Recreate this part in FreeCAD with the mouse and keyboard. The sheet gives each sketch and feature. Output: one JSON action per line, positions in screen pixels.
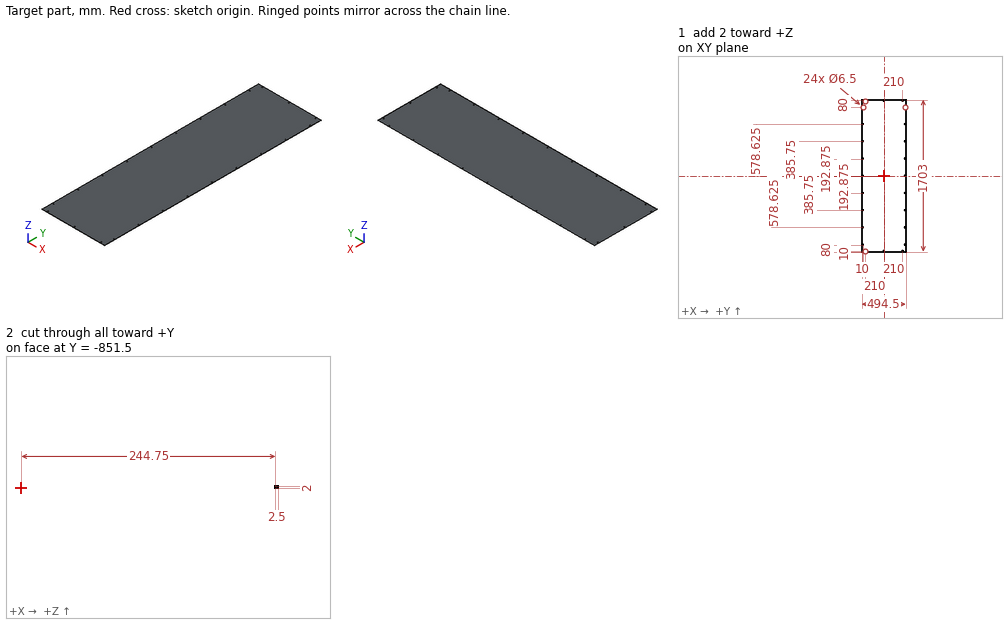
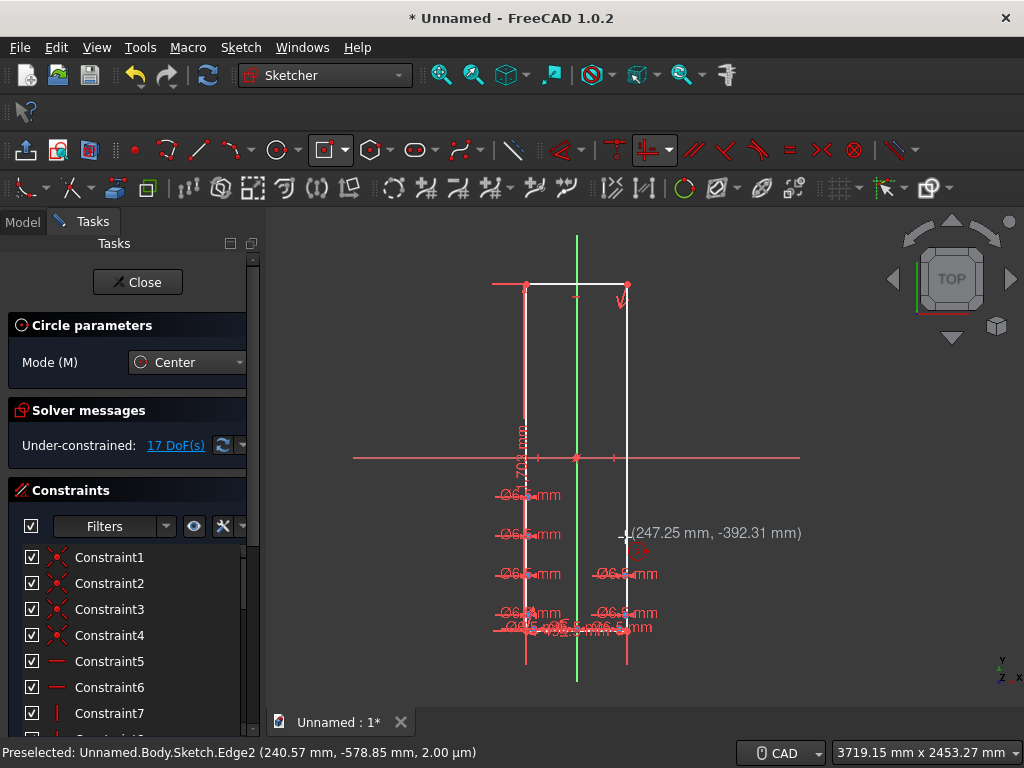
{"action": "scroll", "coordinate": [625, 536], "scroll_direction": "up", "scroll_amount": 11}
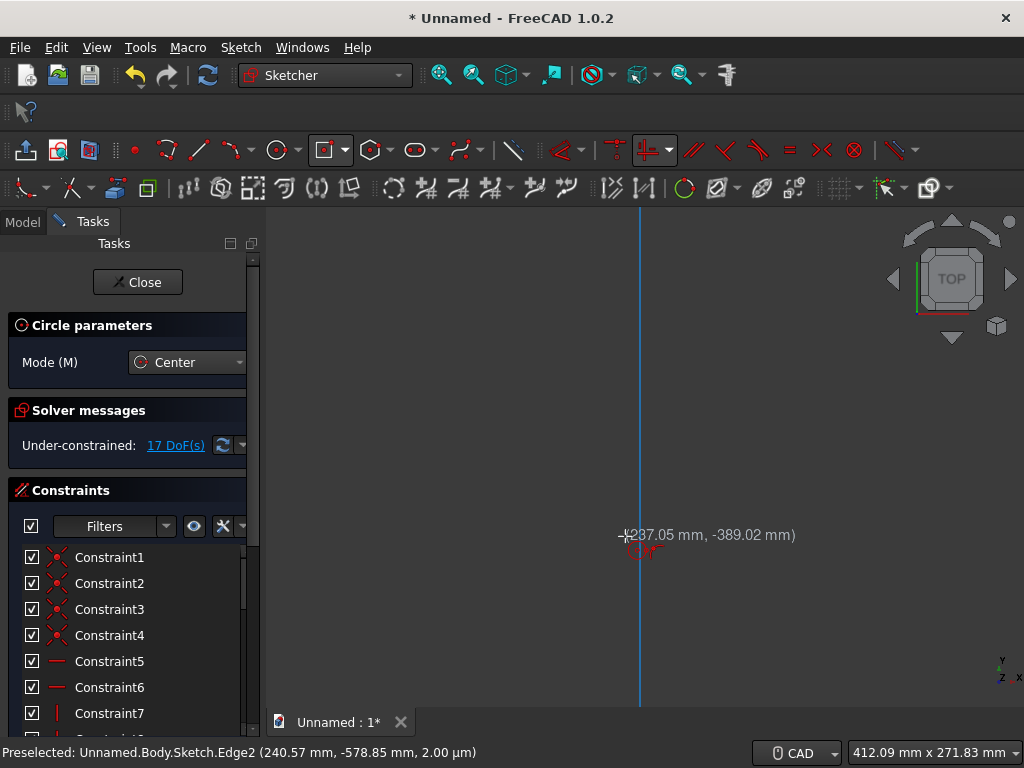
{"action": "left_click", "coordinate": [622, 534]}
{"action": "mouse_move", "coordinate": [626, 529]}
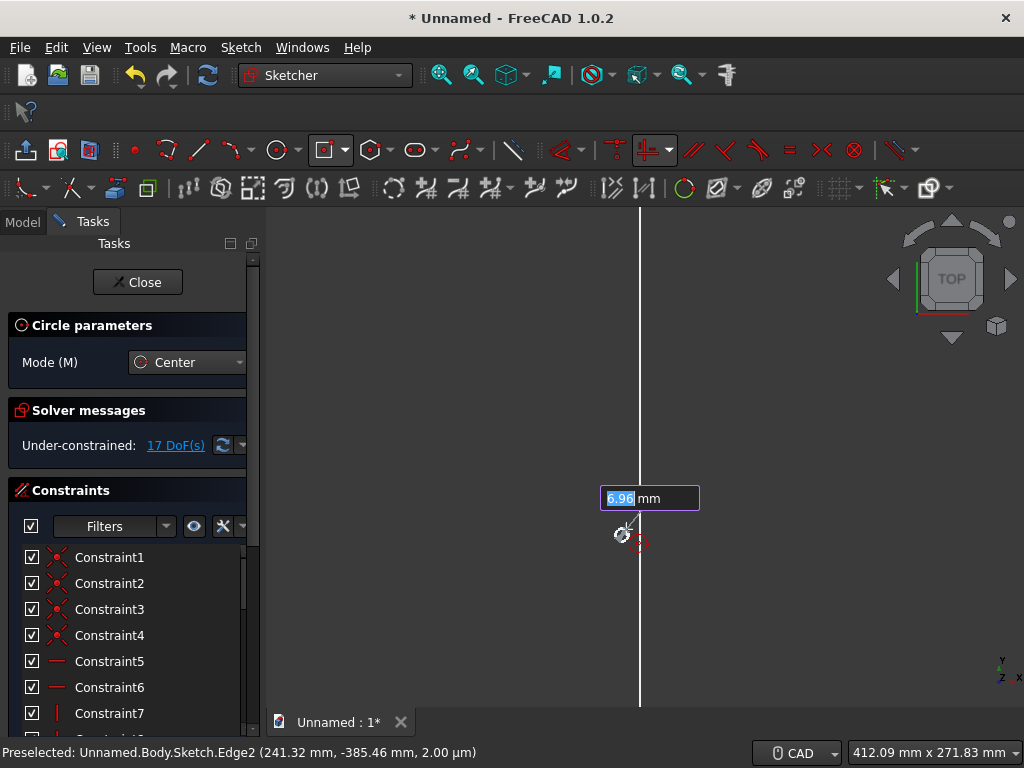
{"action": "type", "text": "6.5"}
{"action": "key", "text": "Return"}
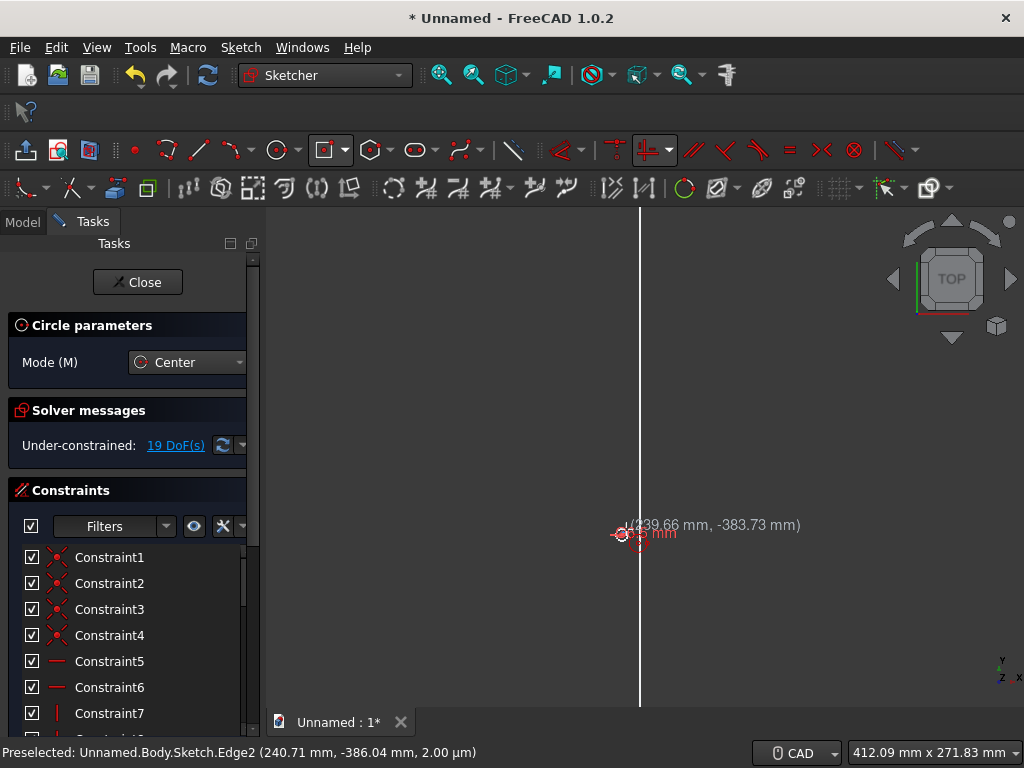
{"action": "scroll", "coordinate": [616, 520], "scroll_direction": "down", "scroll_amount": 12}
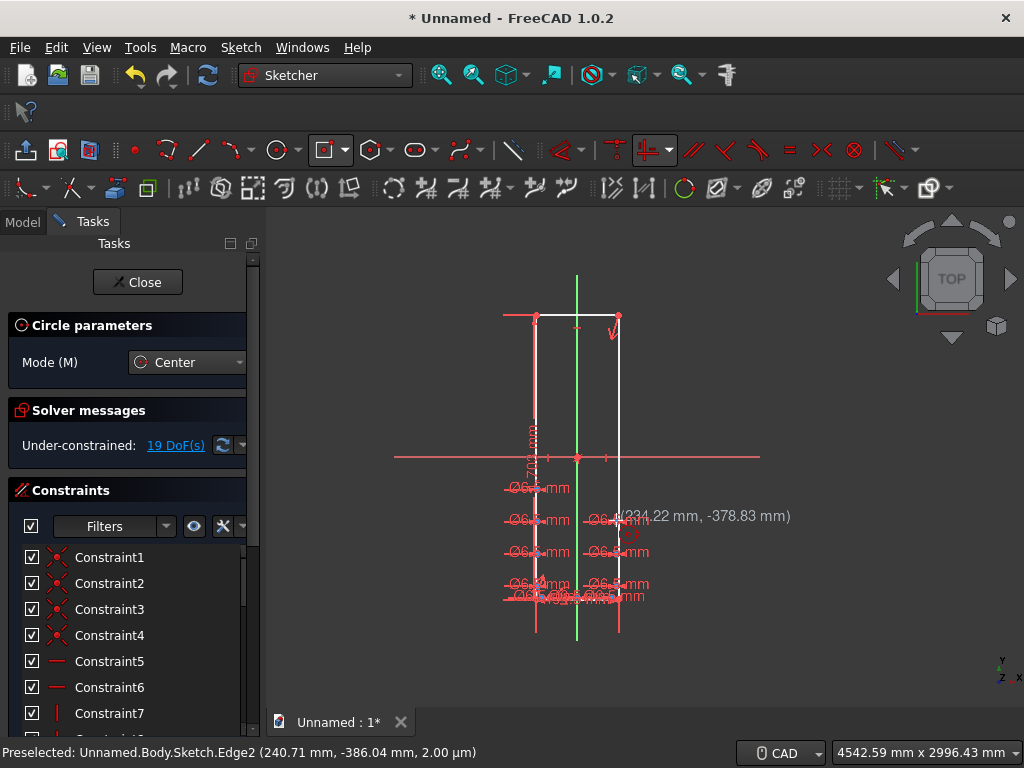
{"action": "scroll", "coordinate": [617, 490], "scroll_direction": "up", "scroll_amount": 19}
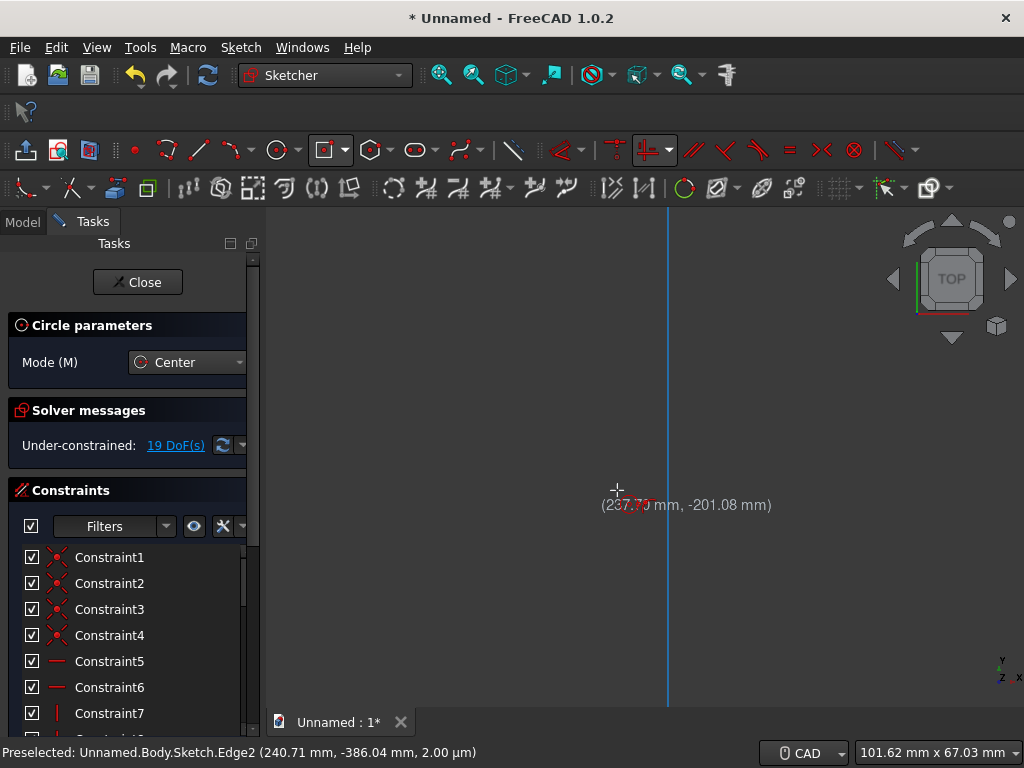
{"action": "scroll", "coordinate": [626, 498], "scroll_direction": "down", "scroll_amount": 18}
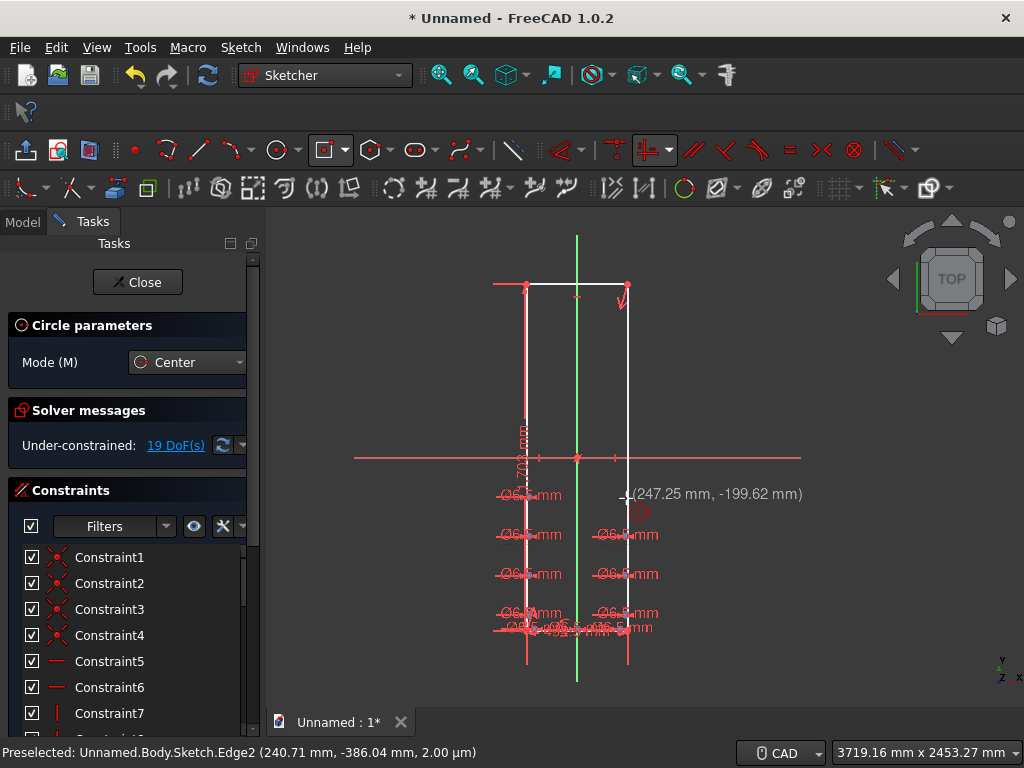
{"action": "scroll", "coordinate": [626, 497], "scroll_direction": "up", "scroll_amount": 11}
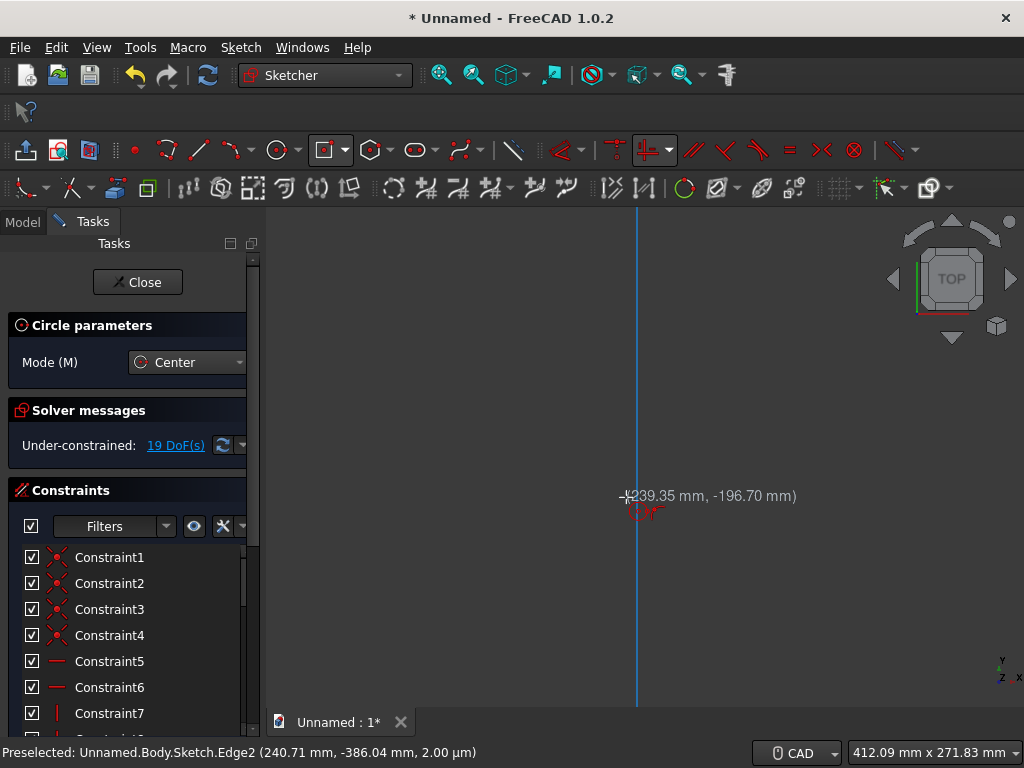
{"action": "left_click", "coordinate": [618, 494]}
{"action": "mouse_move", "coordinate": [623, 490]}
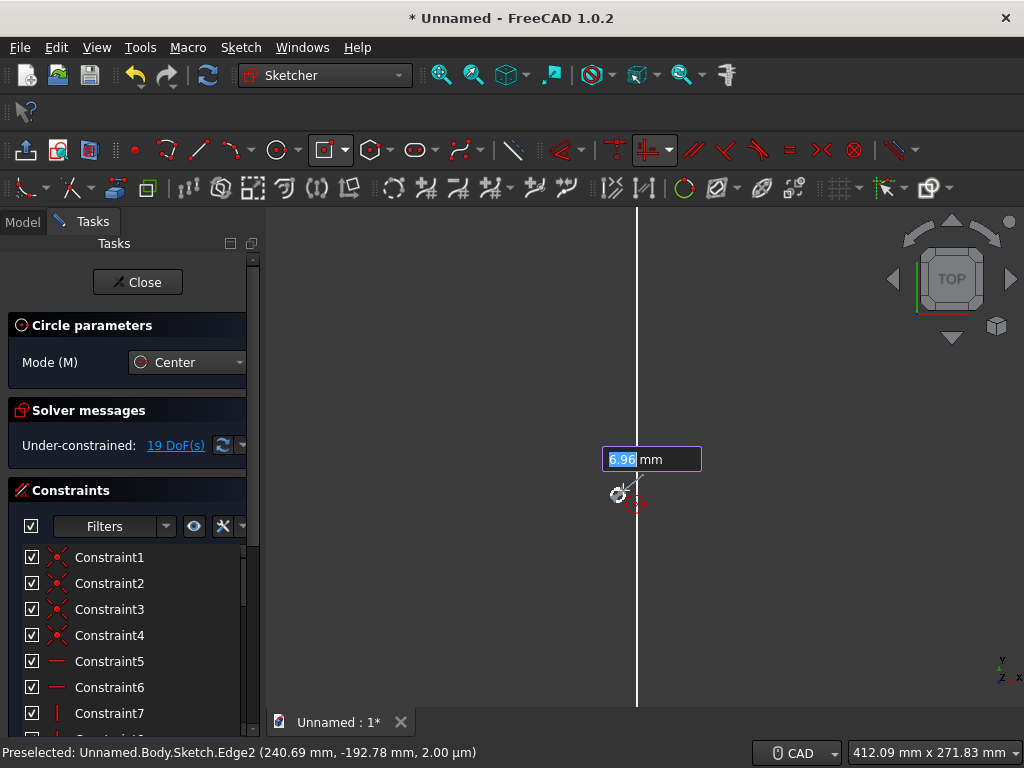
{"action": "type", "text": "6.5"}
{"action": "key", "text": "Return"}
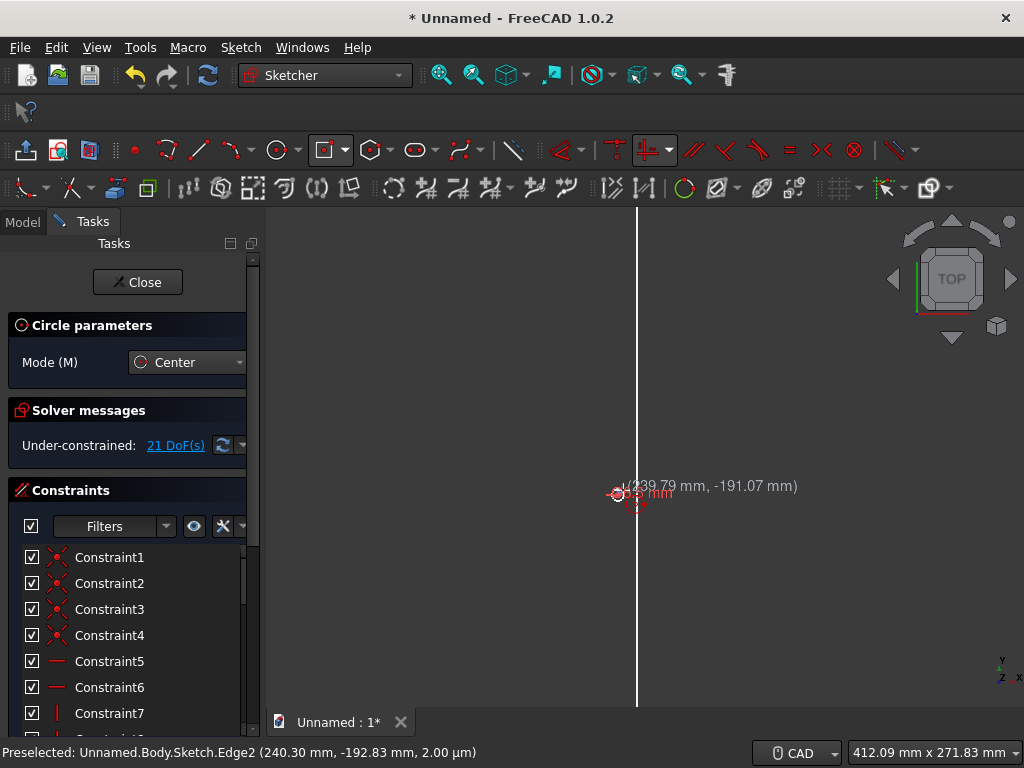
{"action": "scroll", "coordinate": [616, 489], "scroll_direction": "down", "scroll_amount": 12}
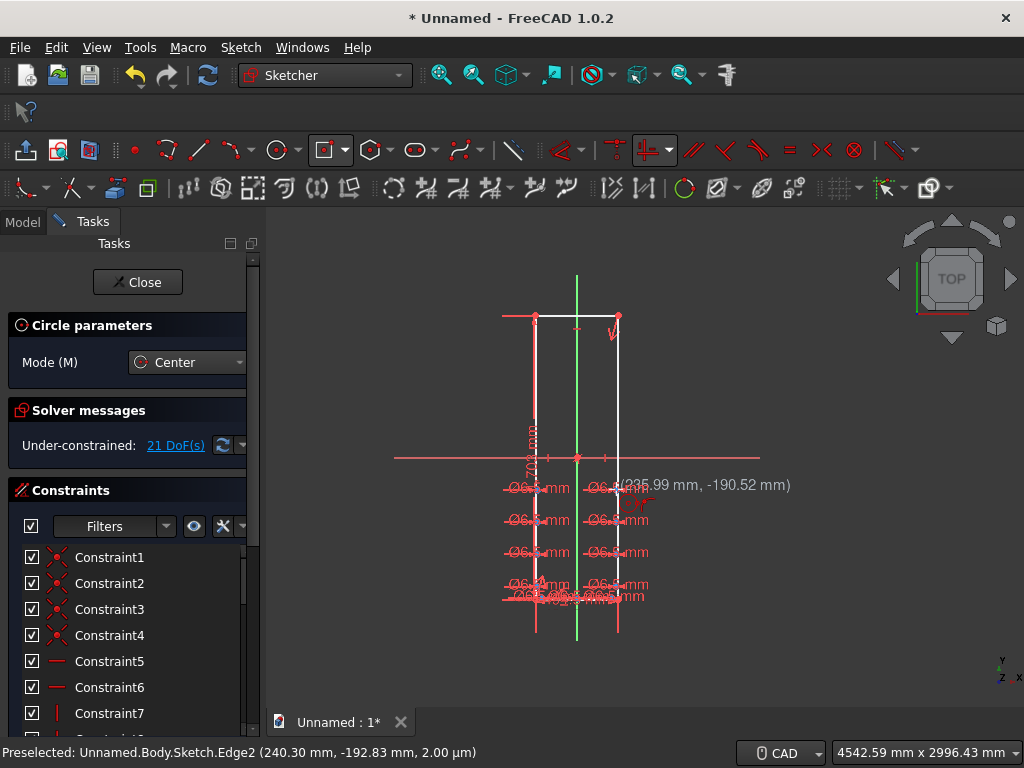
{"action": "scroll", "coordinate": [537, 458], "scroll_direction": "up", "scroll_amount": 19}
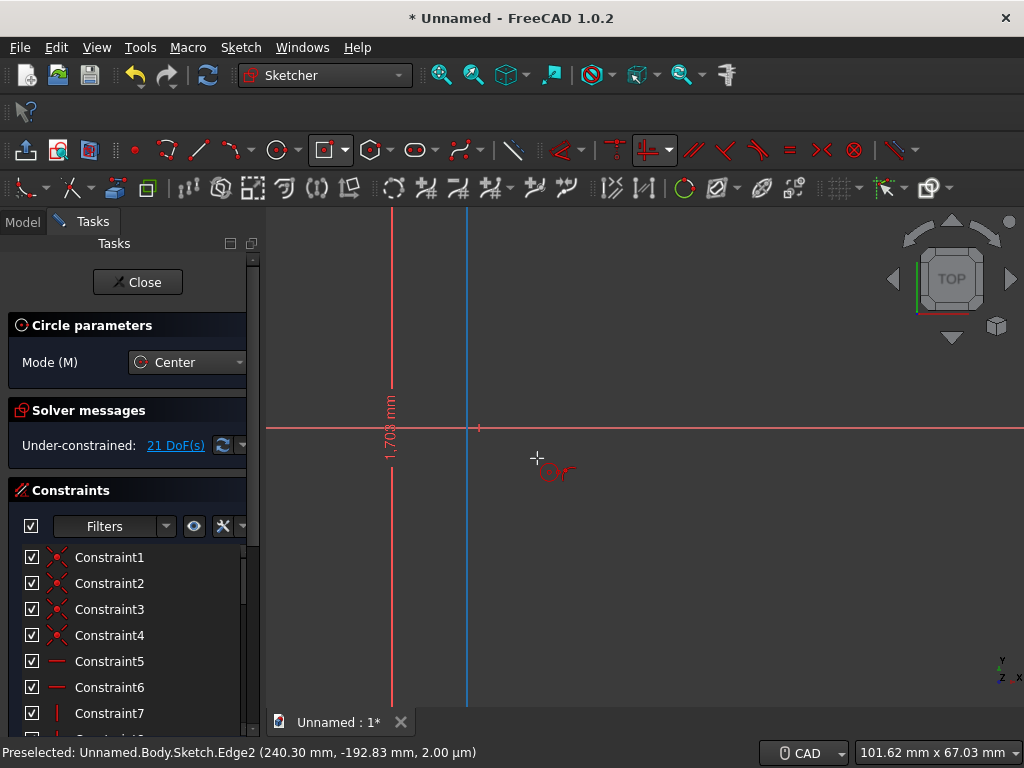
{"action": "scroll", "coordinate": [528, 458], "scroll_direction": "down", "scroll_amount": 18}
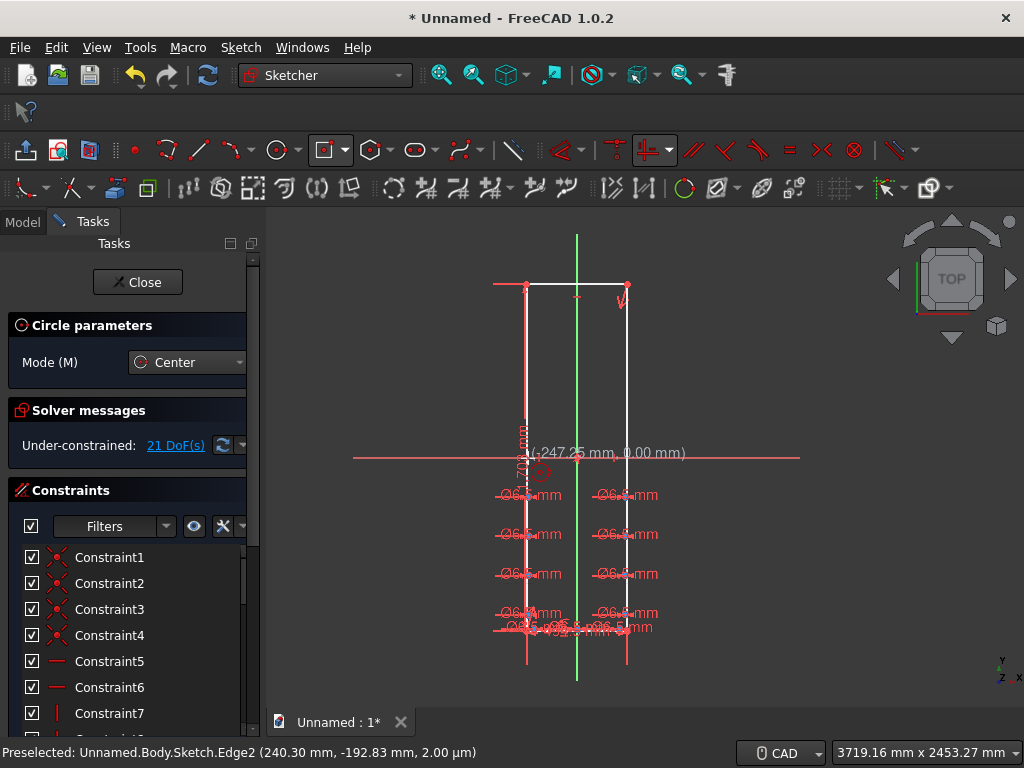
{"action": "scroll", "coordinate": [529, 458], "scroll_direction": "up", "scroll_amount": 11}